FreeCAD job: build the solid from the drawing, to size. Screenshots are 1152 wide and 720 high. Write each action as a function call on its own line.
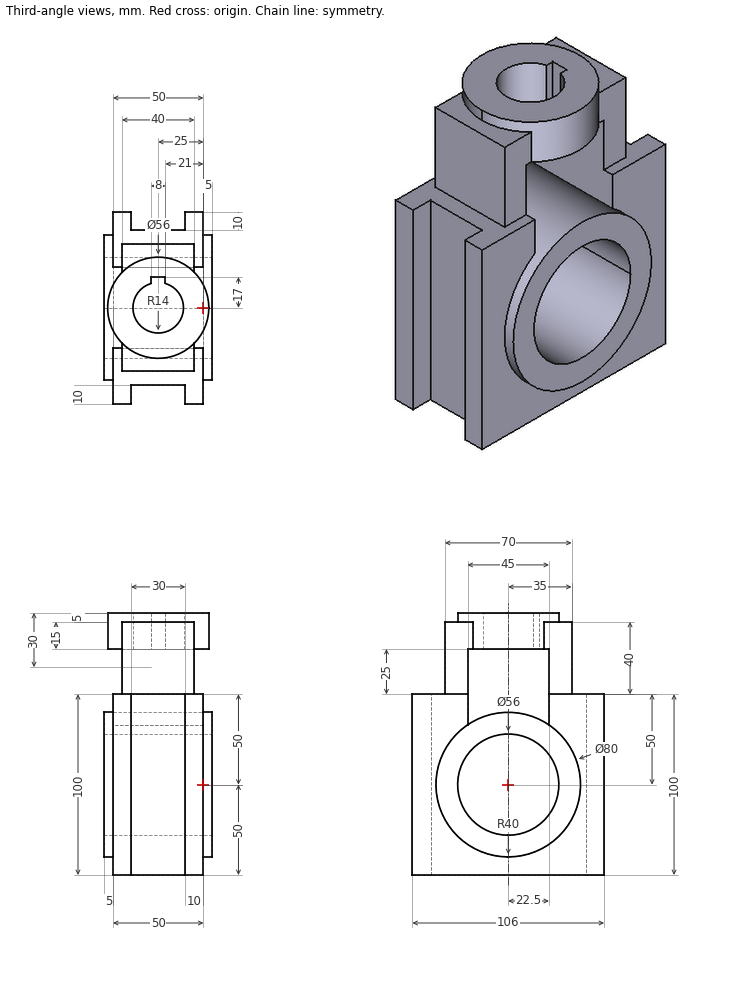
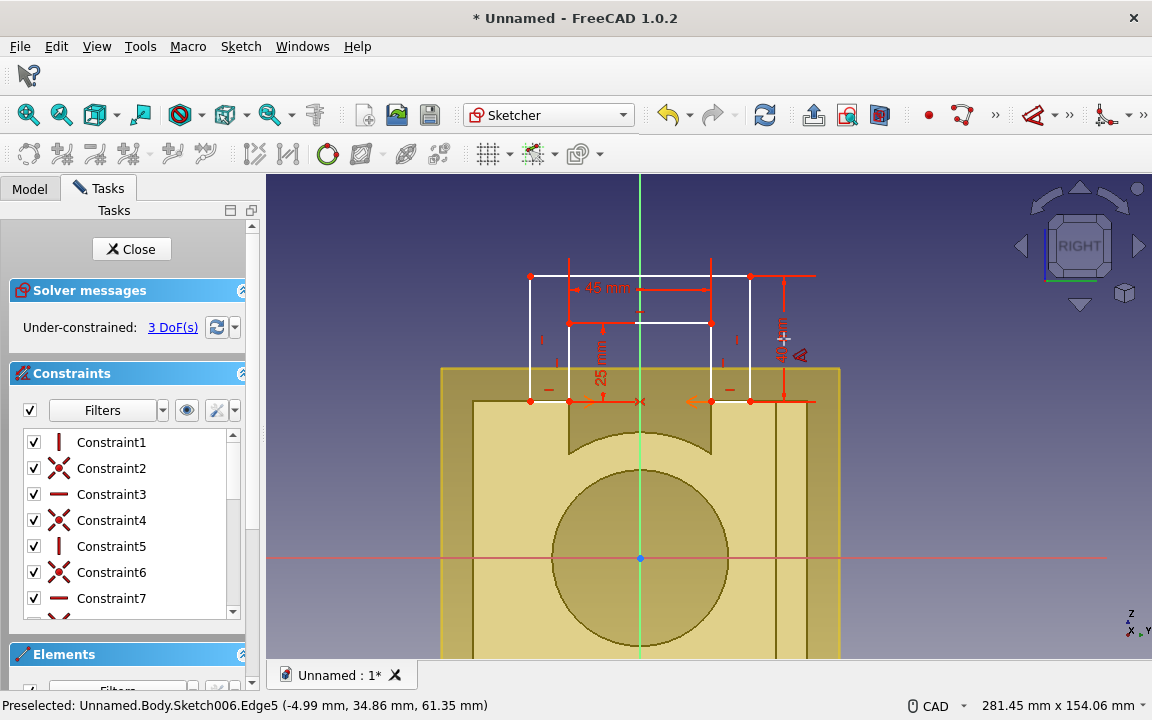
click(684, 276)
click(589, 242)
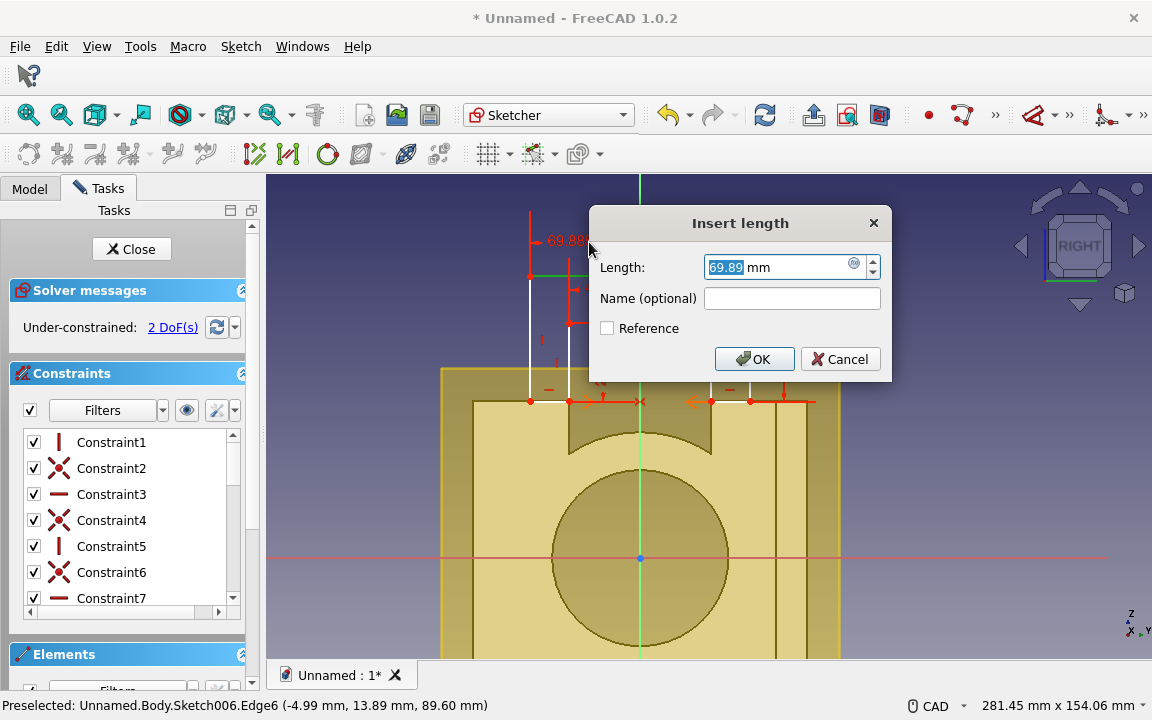
text(70)
key(Return)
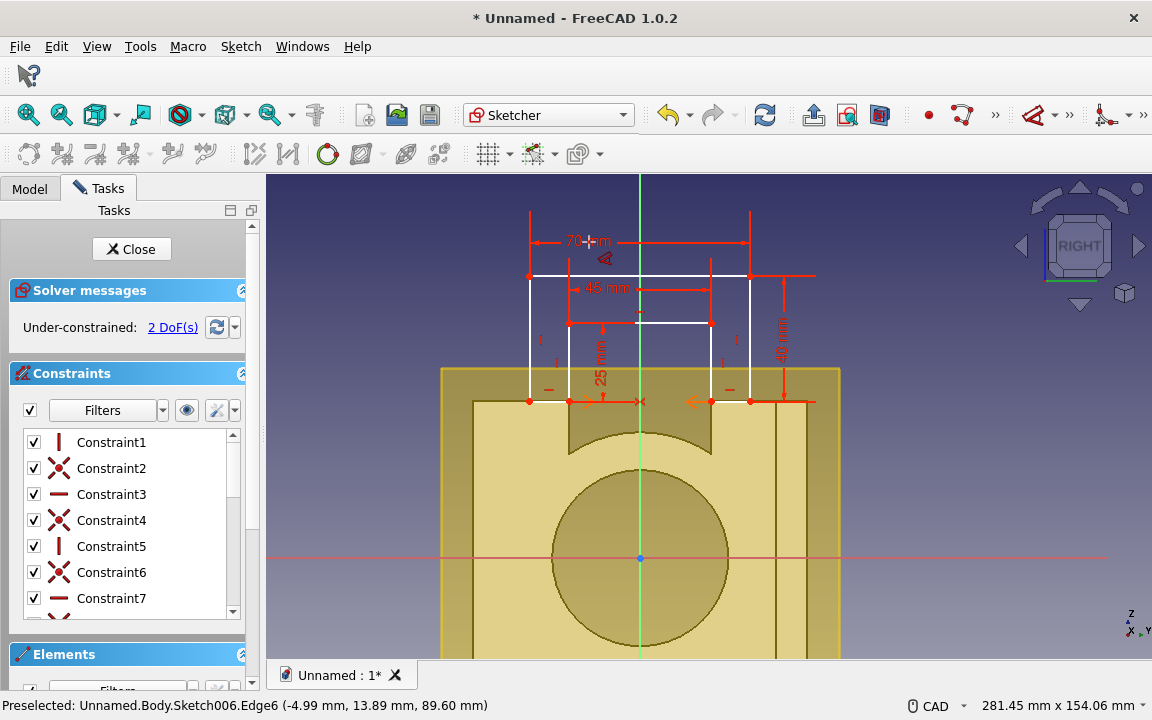
click(569, 402)
click(535, 480)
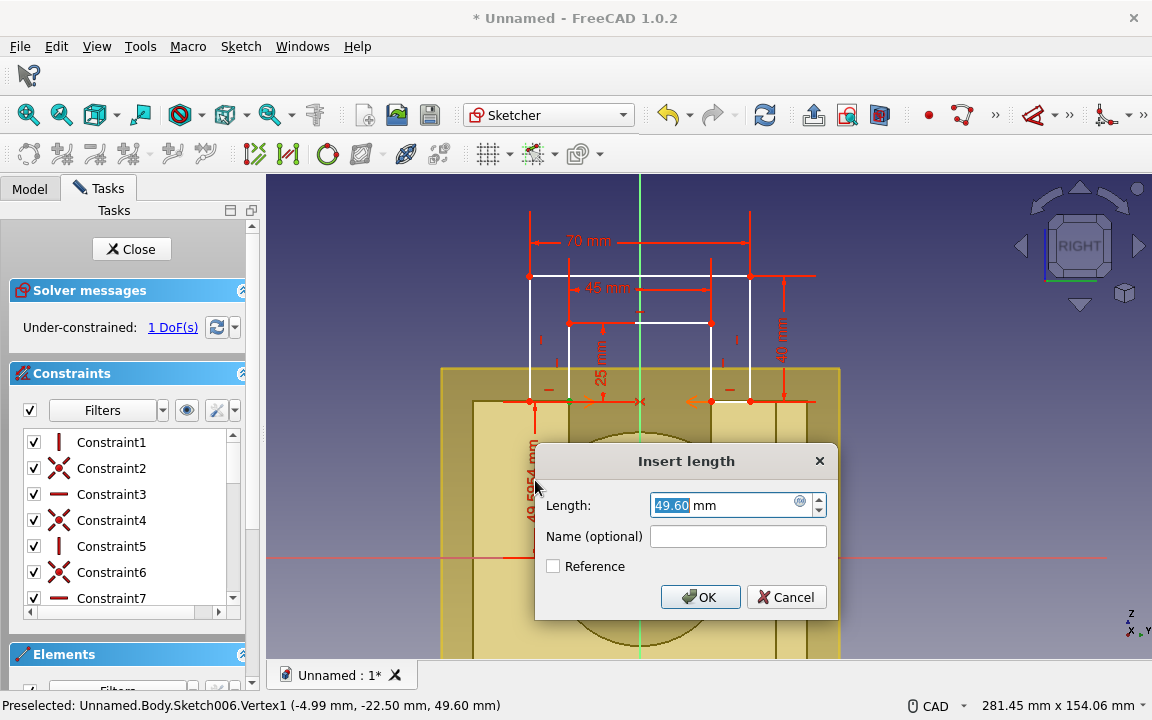
text(50)
key(Return)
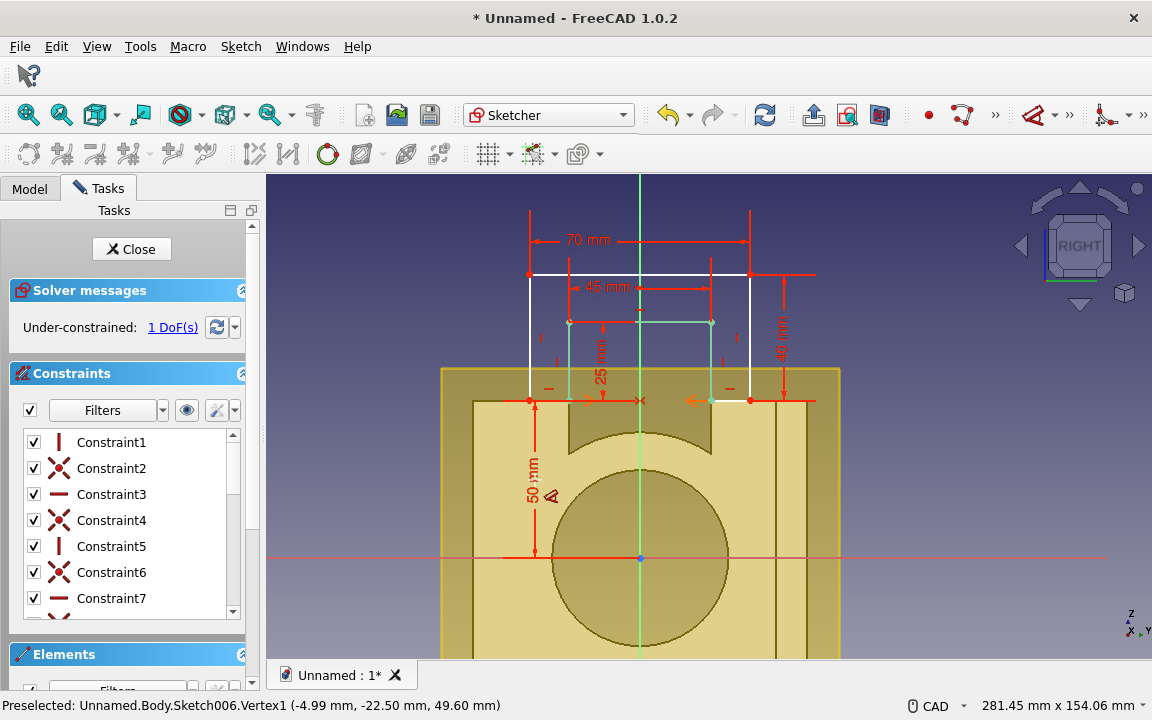
click(750, 401)
click(695, 592)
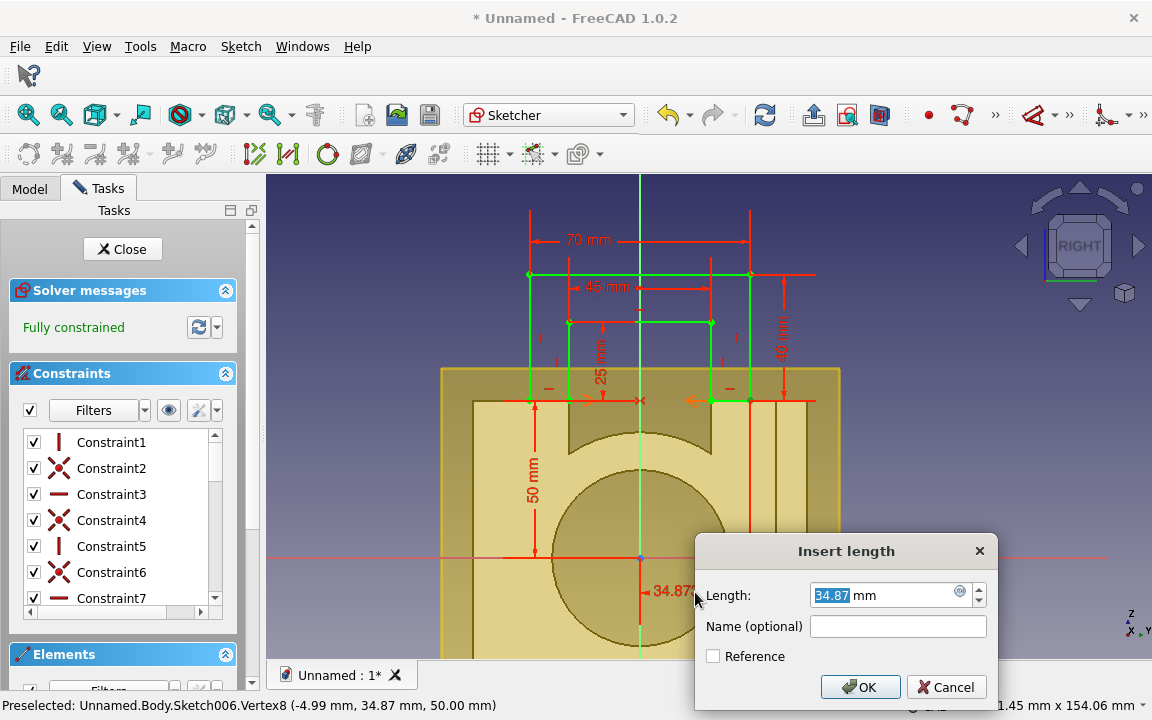
text(35)
key(Return)
key(Escape)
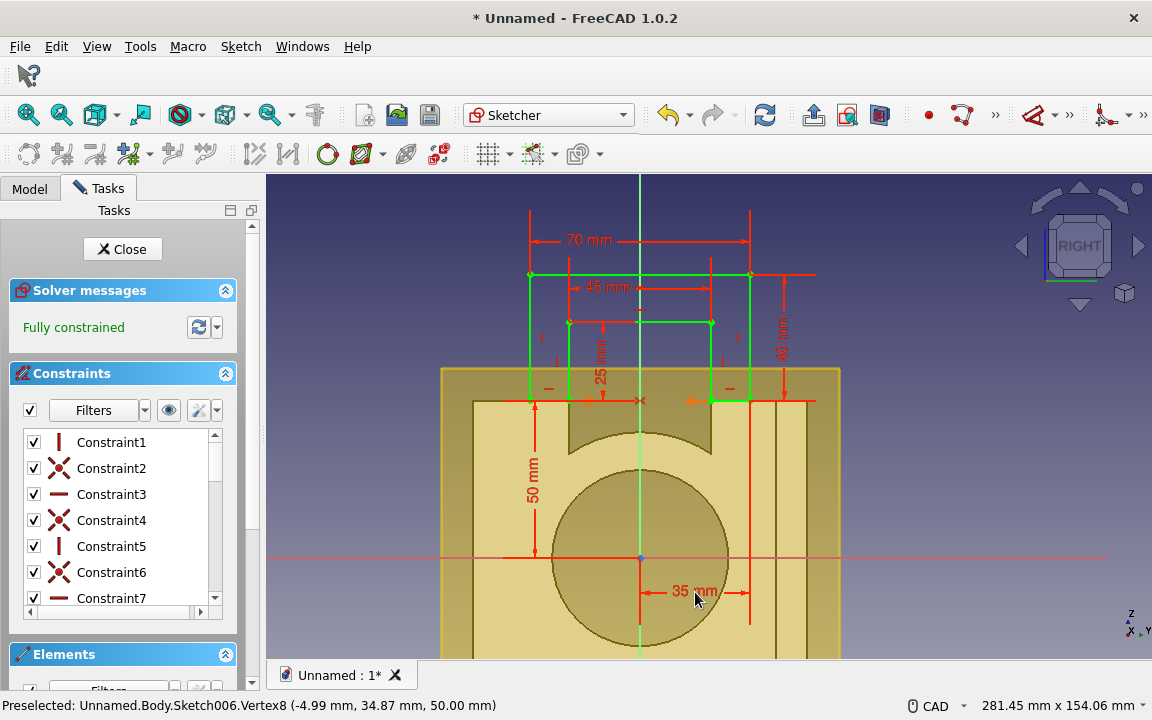
click(123, 249)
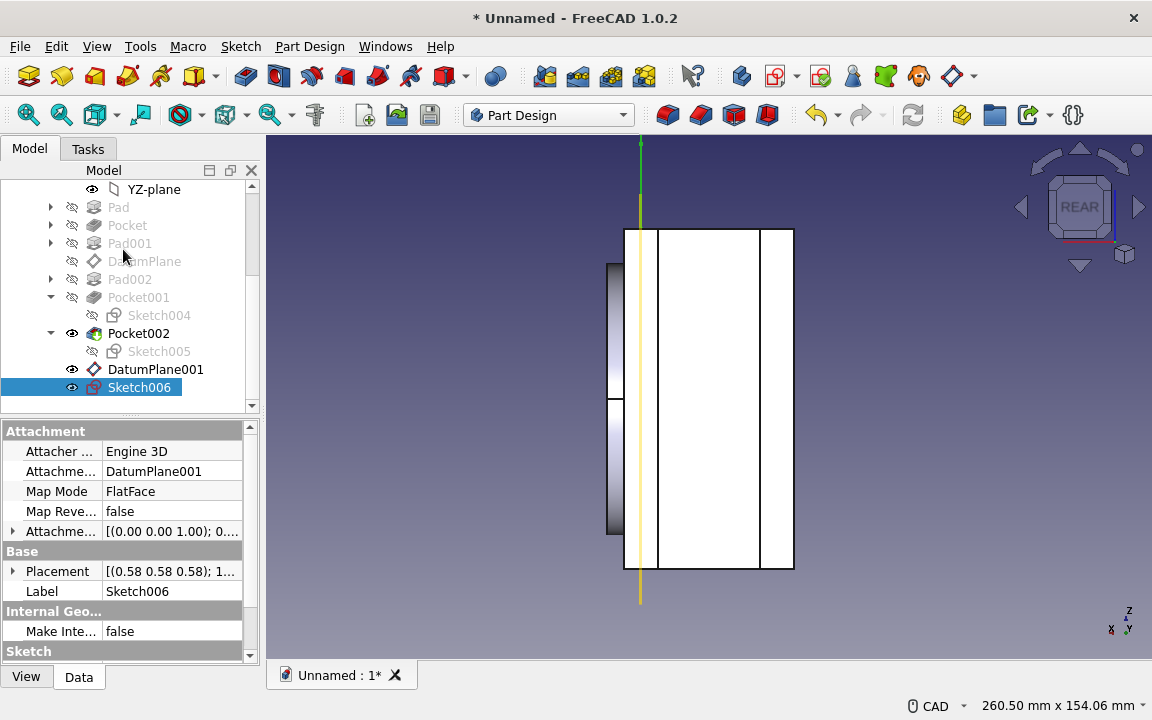
click(29, 76)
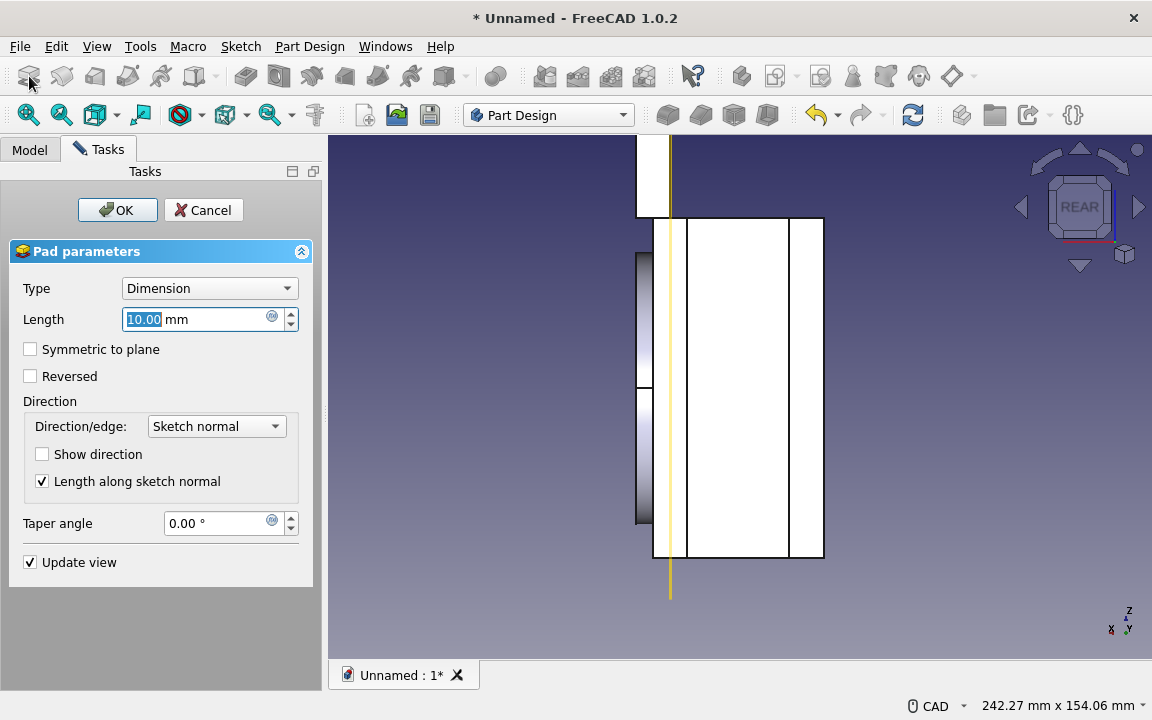
text(40)
key(Tab)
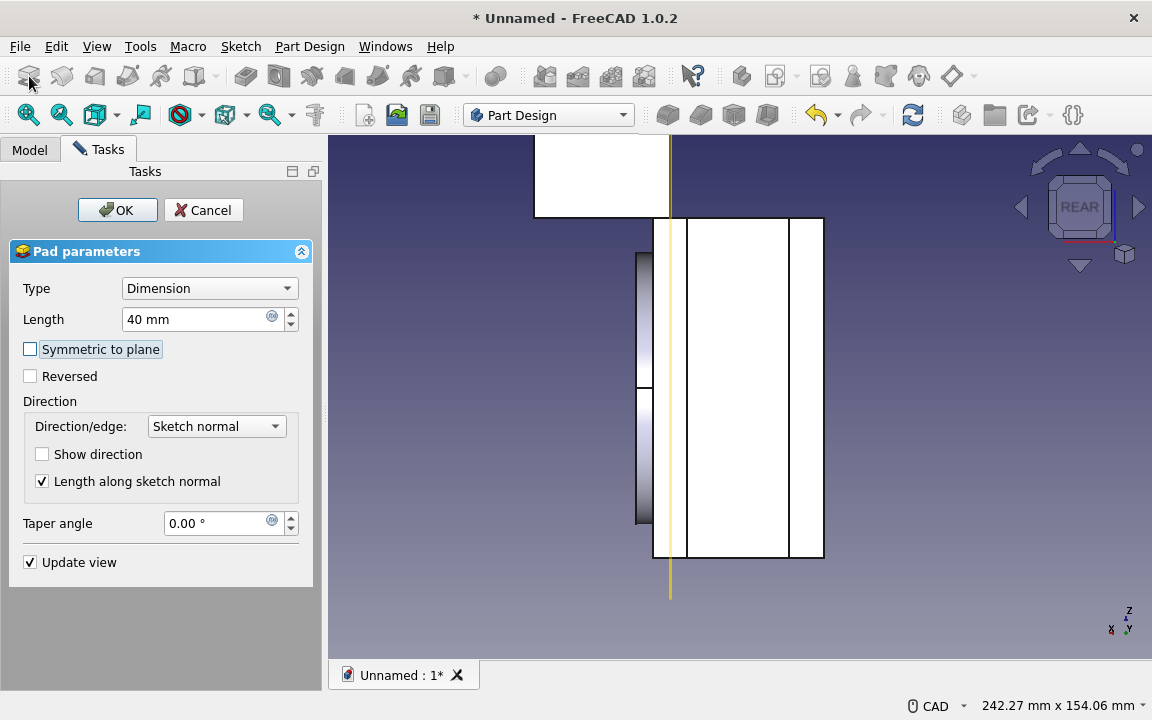
click(31, 376)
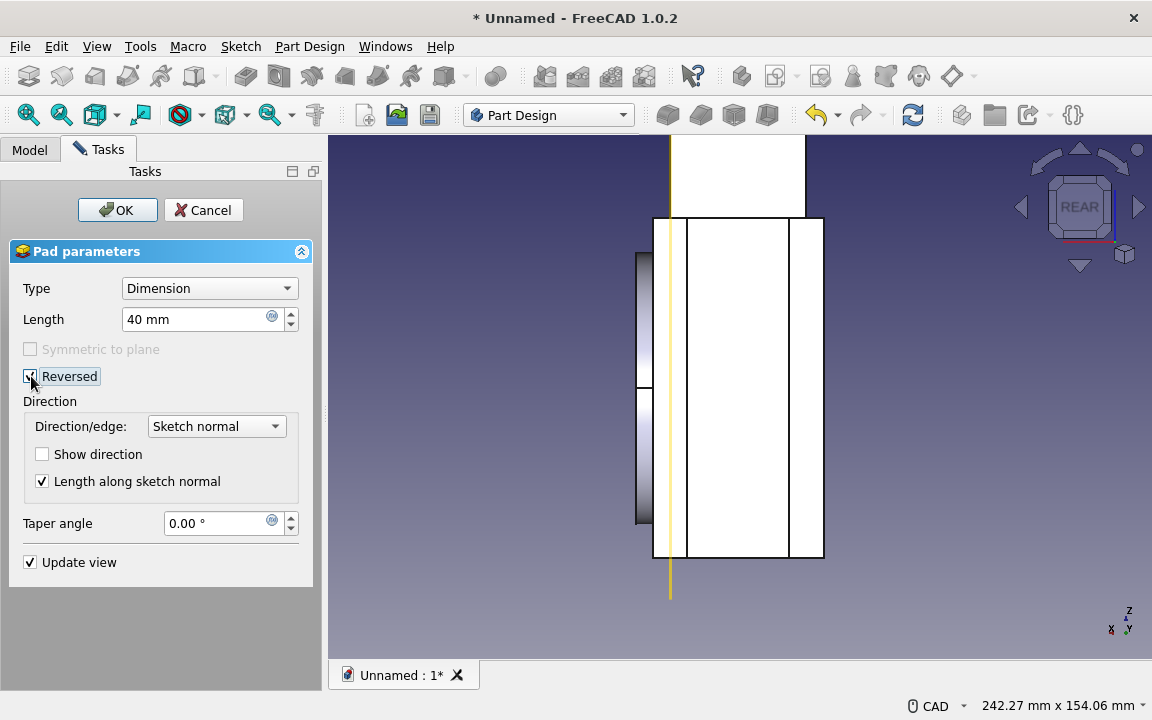
click(118, 210)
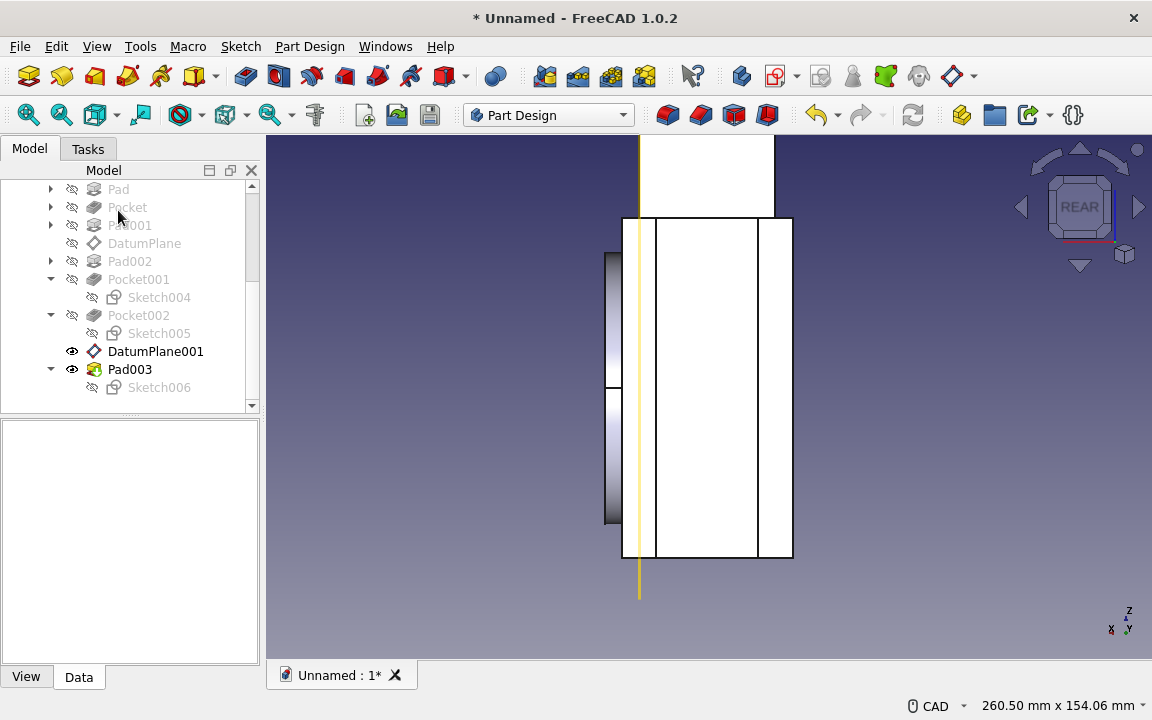
click(117, 351)
key(space)